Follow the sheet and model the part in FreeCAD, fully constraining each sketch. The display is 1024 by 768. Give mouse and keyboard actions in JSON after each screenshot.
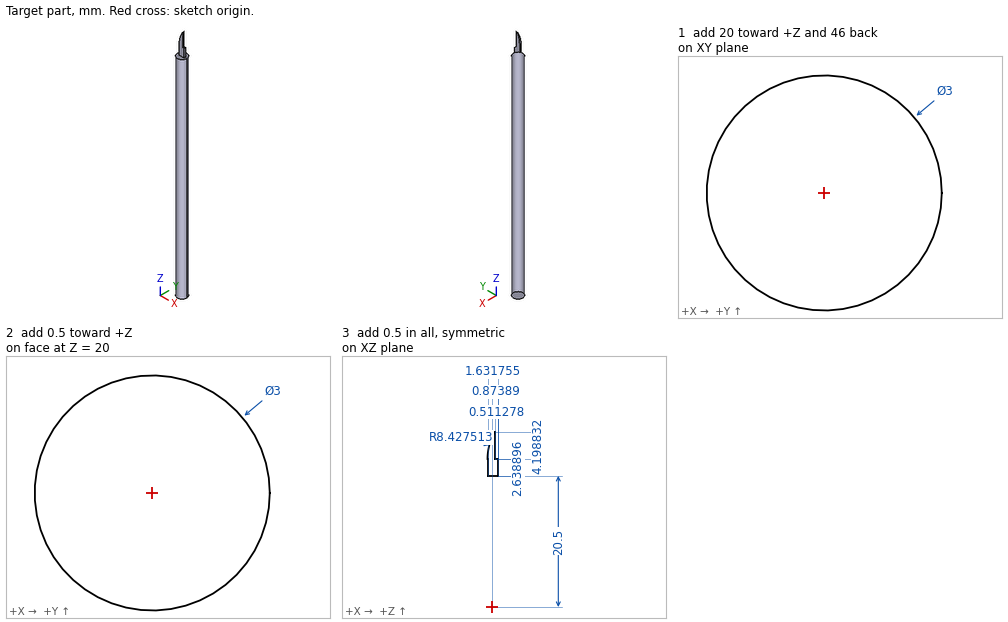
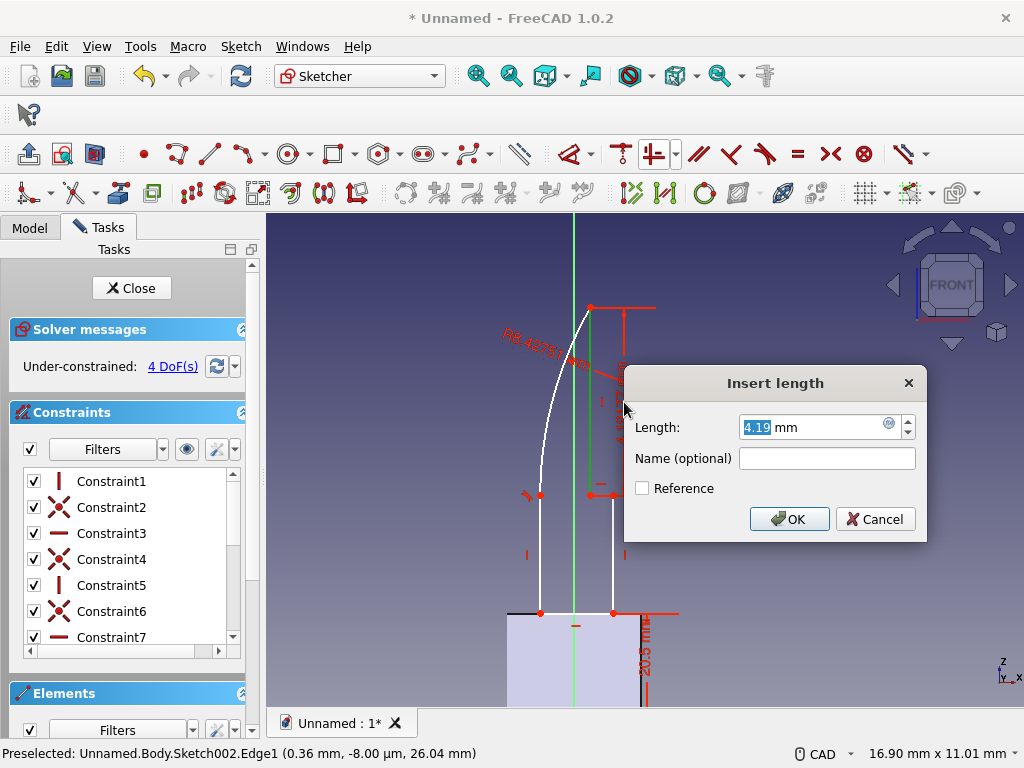
{"action": "type", "text": "4.198832"}
{"action": "key", "text": "Return"}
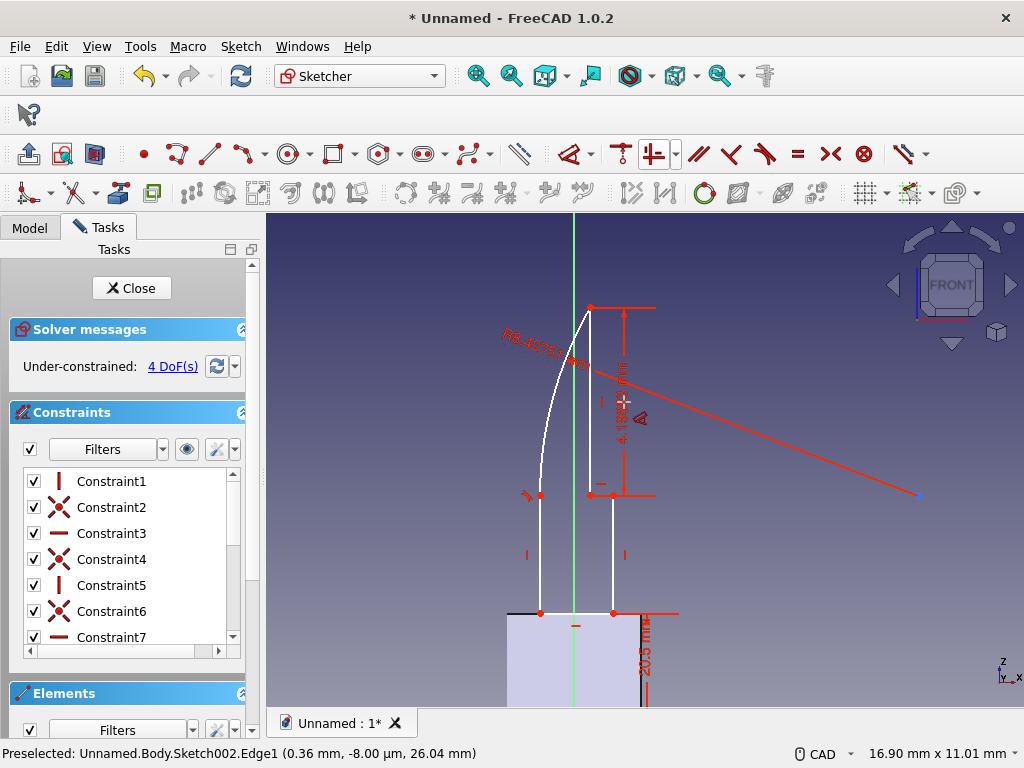
{"action": "scroll", "coordinate": [600, 496], "scroll_direction": "up", "scroll_amount": 3}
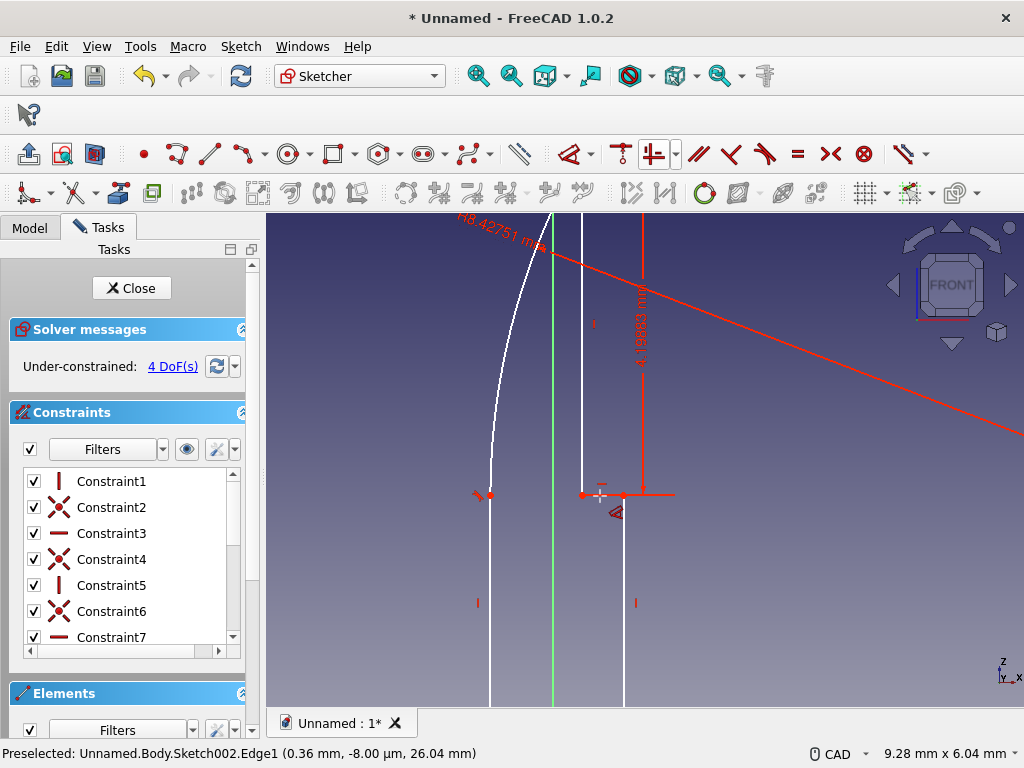
{"action": "left_click", "coordinate": [599, 495]}
{"action": "left_click", "coordinate": [603, 529]}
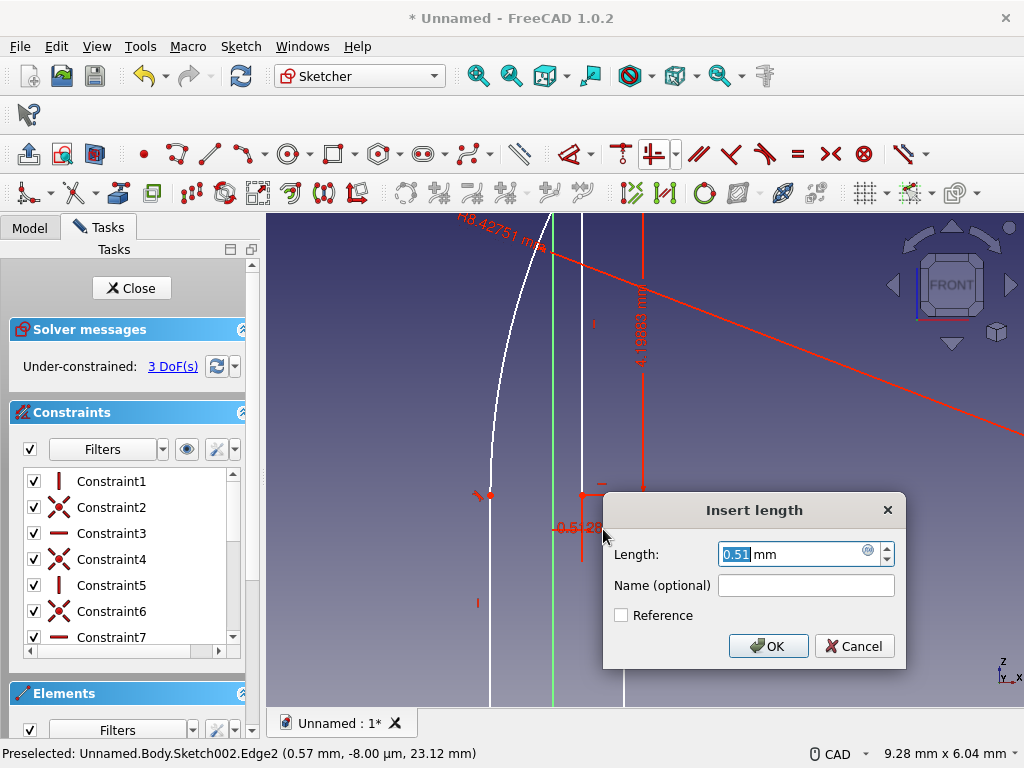
{"action": "type", "text": "0.511278"}
{"action": "key", "text": "Return"}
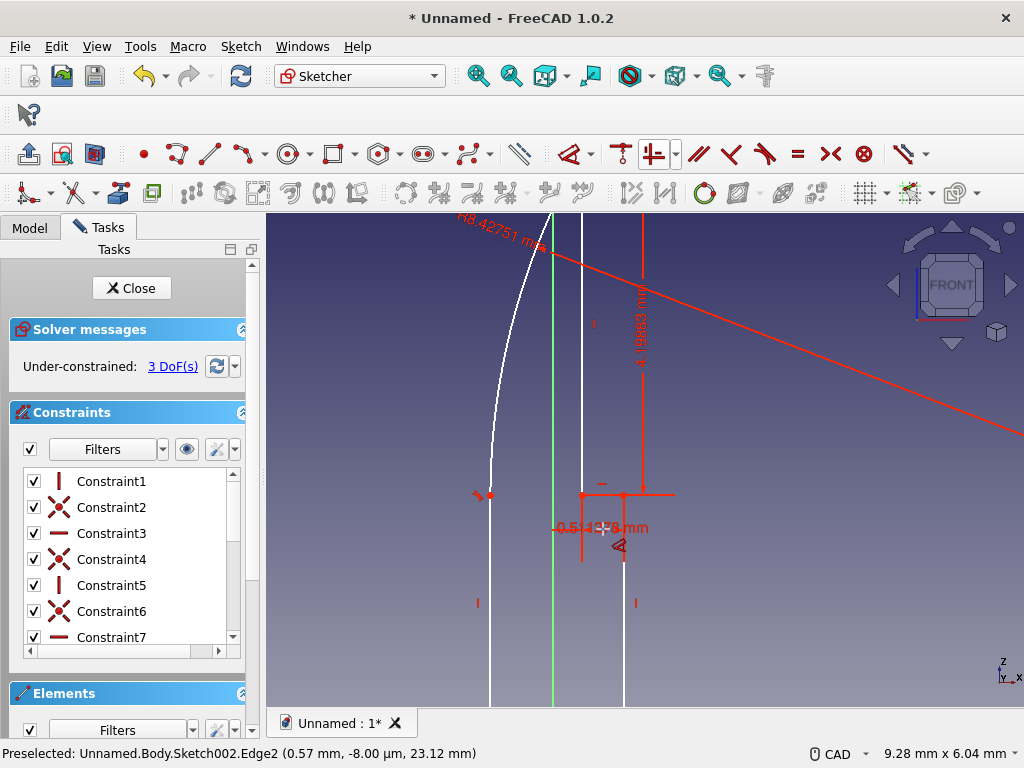
{"action": "left_click", "coordinate": [624, 560]}
{"action": "left_click", "coordinate": [658, 587]}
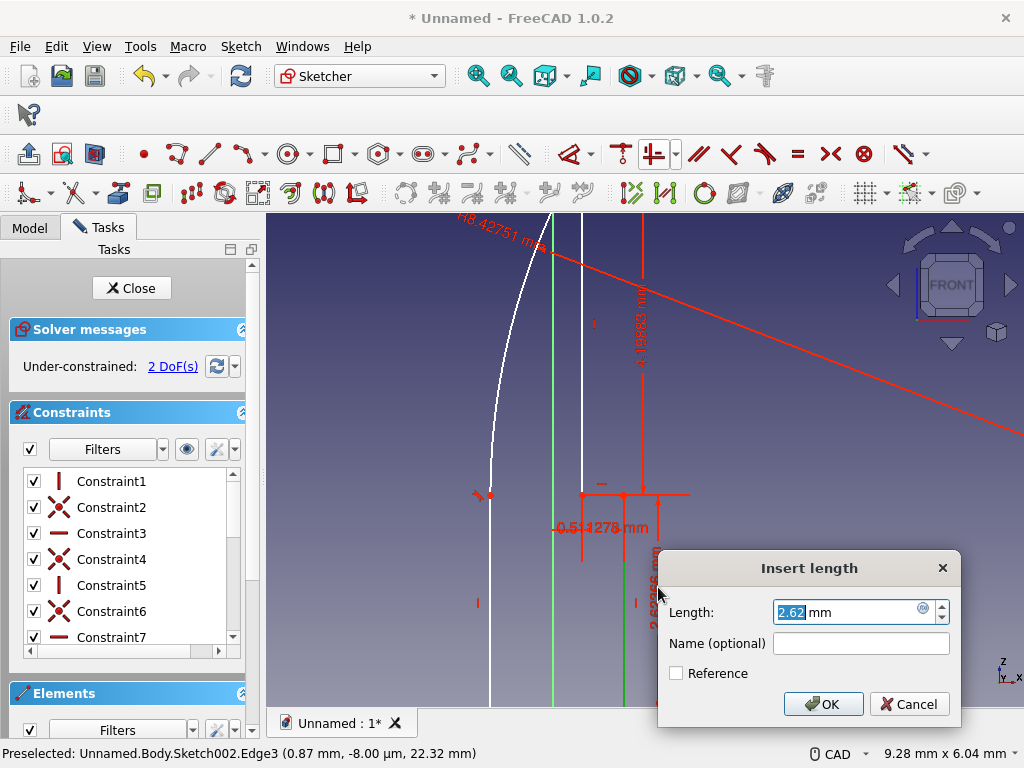
{"action": "type", "text": "2.638896"}
{"action": "key", "text": "Return"}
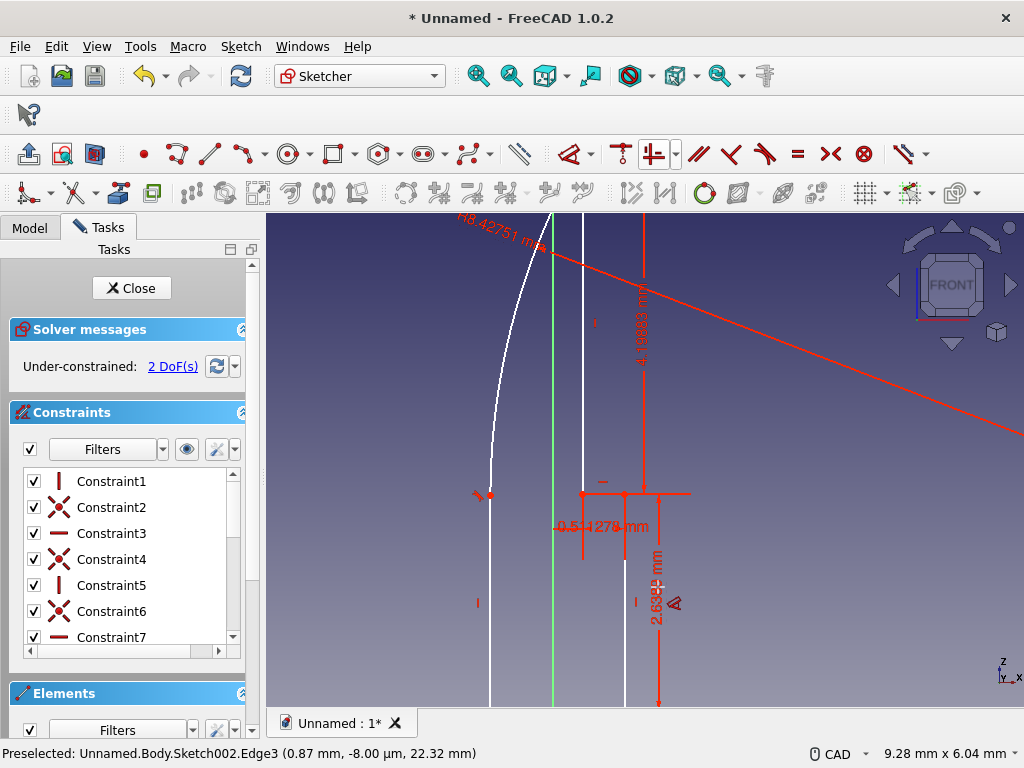
{"action": "scroll", "coordinate": [600, 496], "scroll_direction": "down", "scroll_amount": 3}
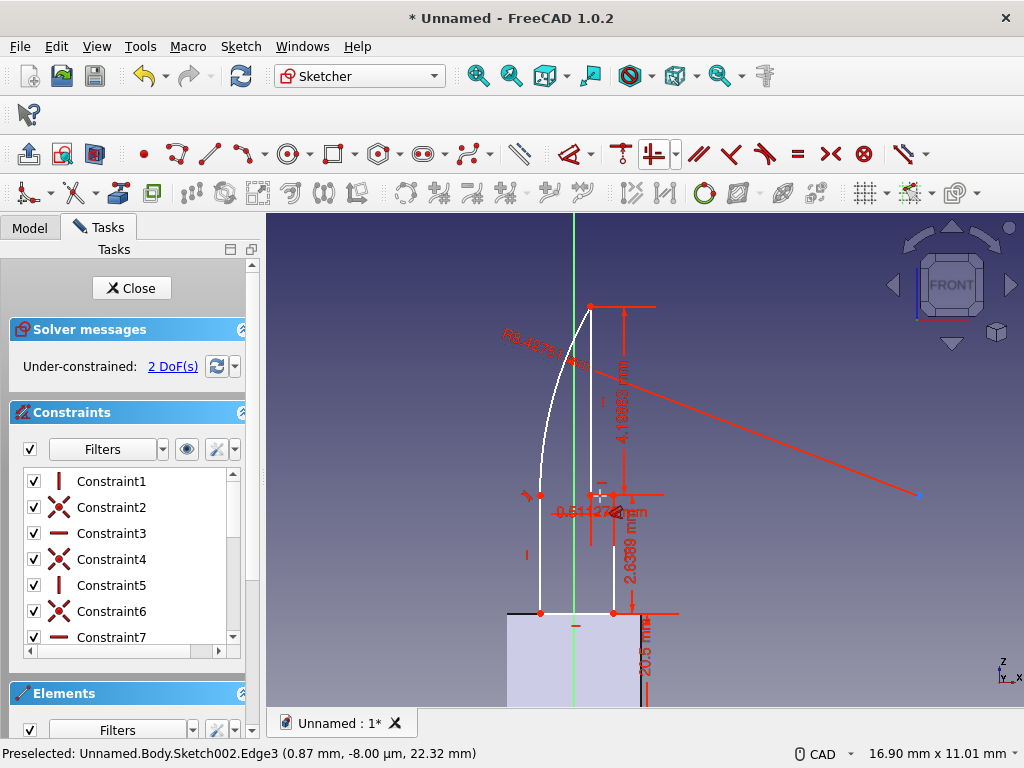
{"action": "left_click", "coordinate": [592, 614]}
{"action": "left_click", "coordinate": [560, 648]}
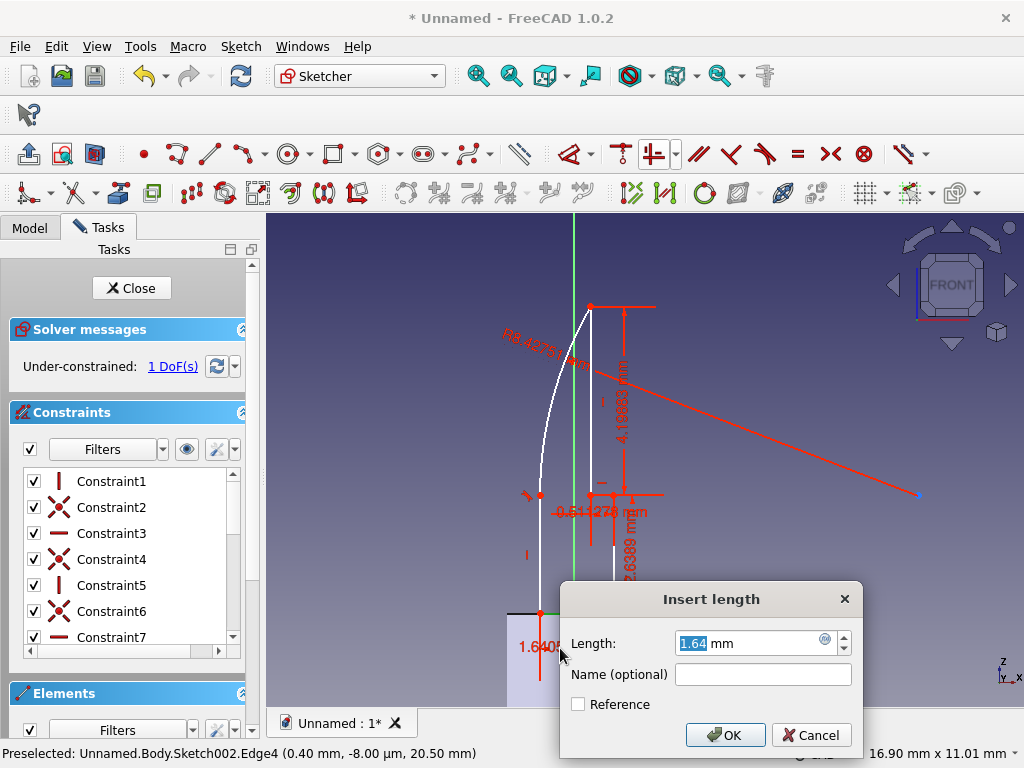
{"action": "type", "text": "1.631755"}
{"action": "key", "text": "Return"}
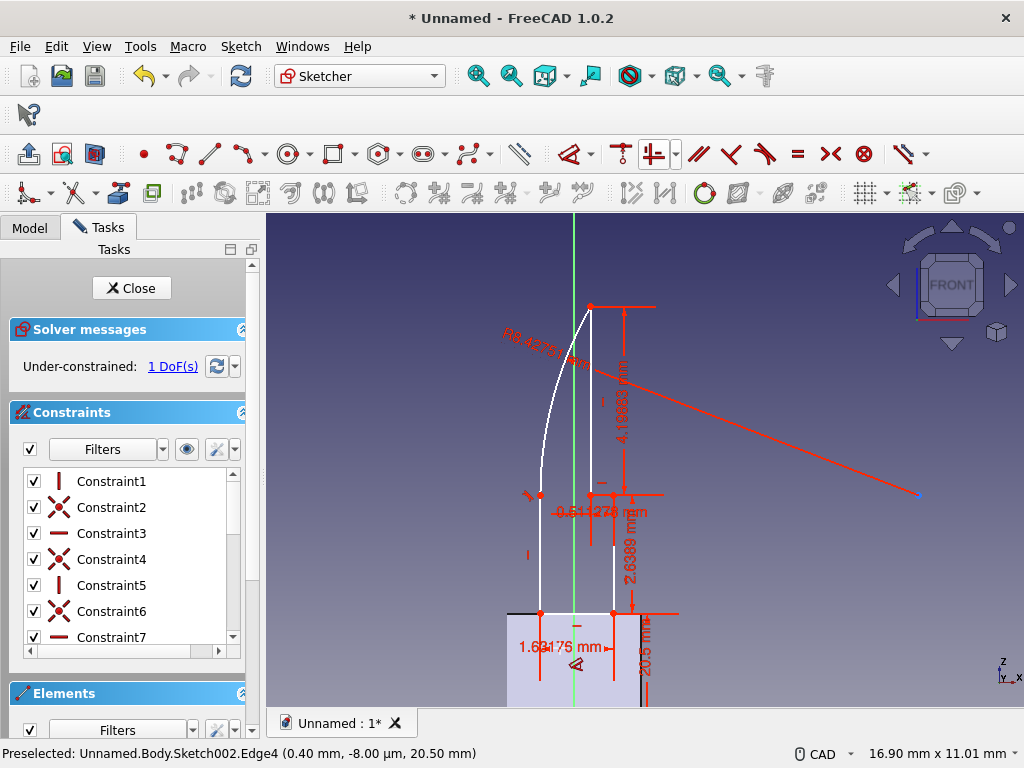
{"action": "left_click", "coordinate": [614, 495]}
{"action": "left_click", "coordinate": [608, 461]}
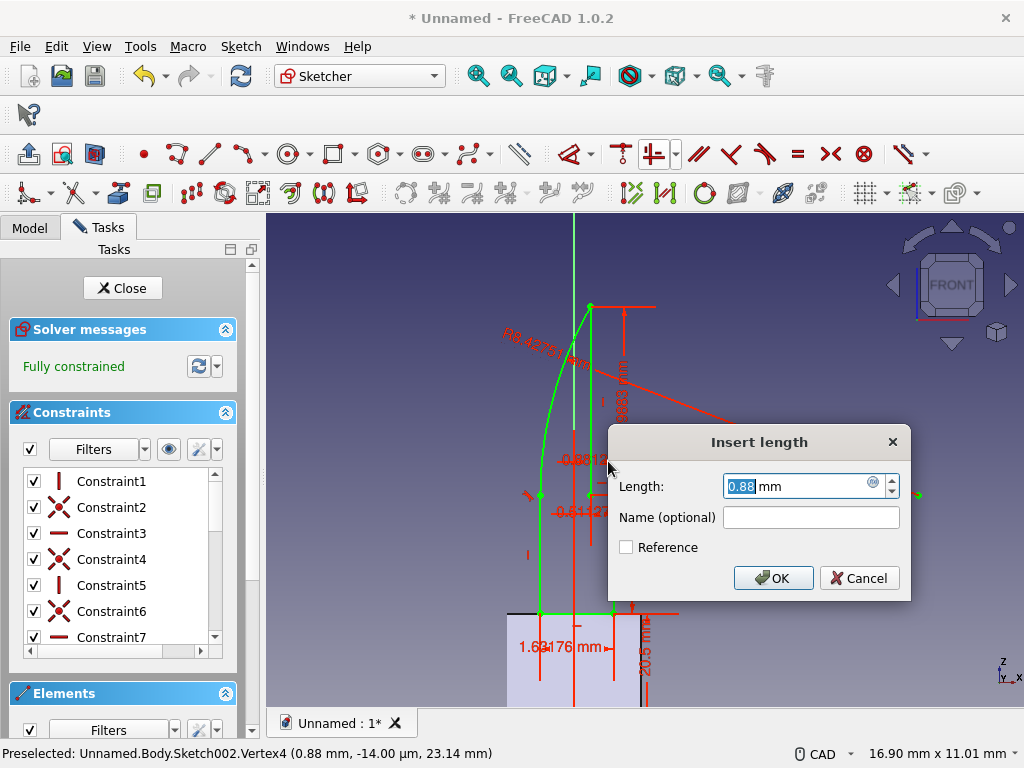
{"action": "type", "text": "0.87389"}
{"action": "key", "text": "Return"}
{"action": "key", "text": "Escape"}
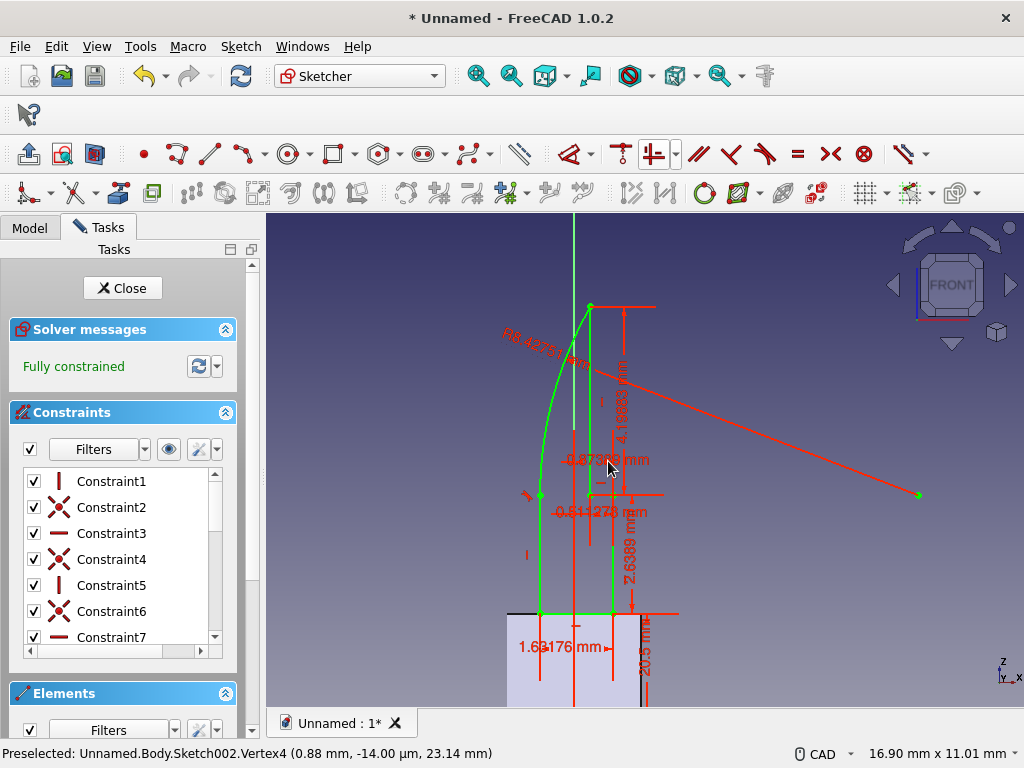
{"action": "left_click", "coordinate": [123, 288]}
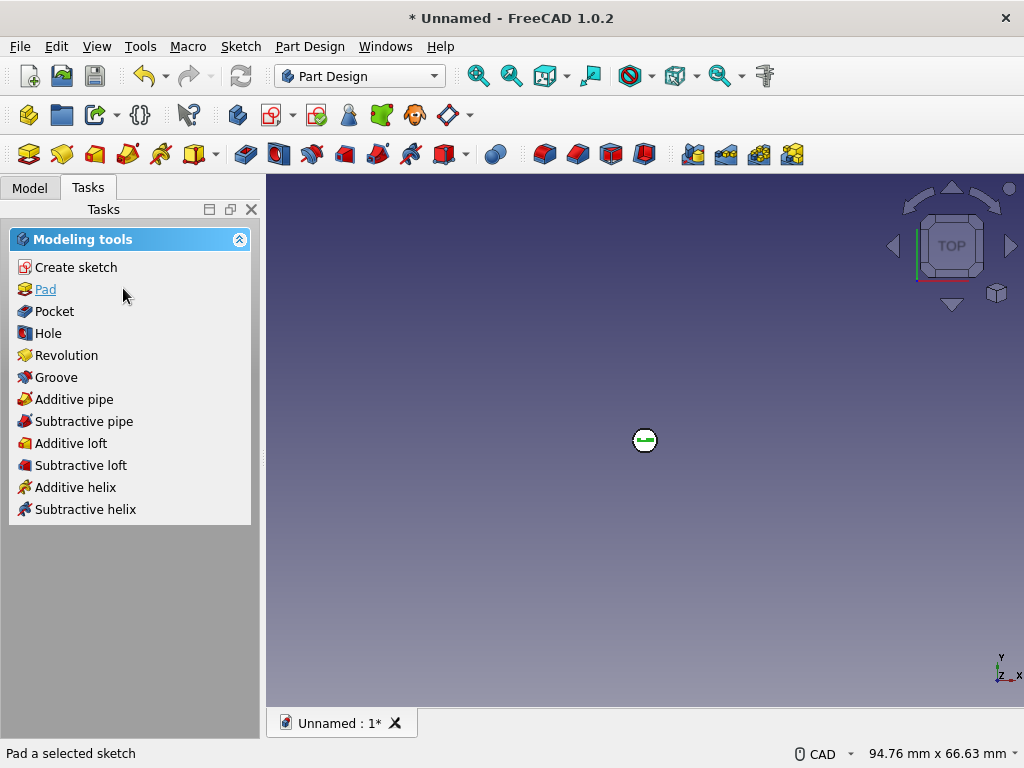
{"action": "left_click", "coordinate": [29, 154]}